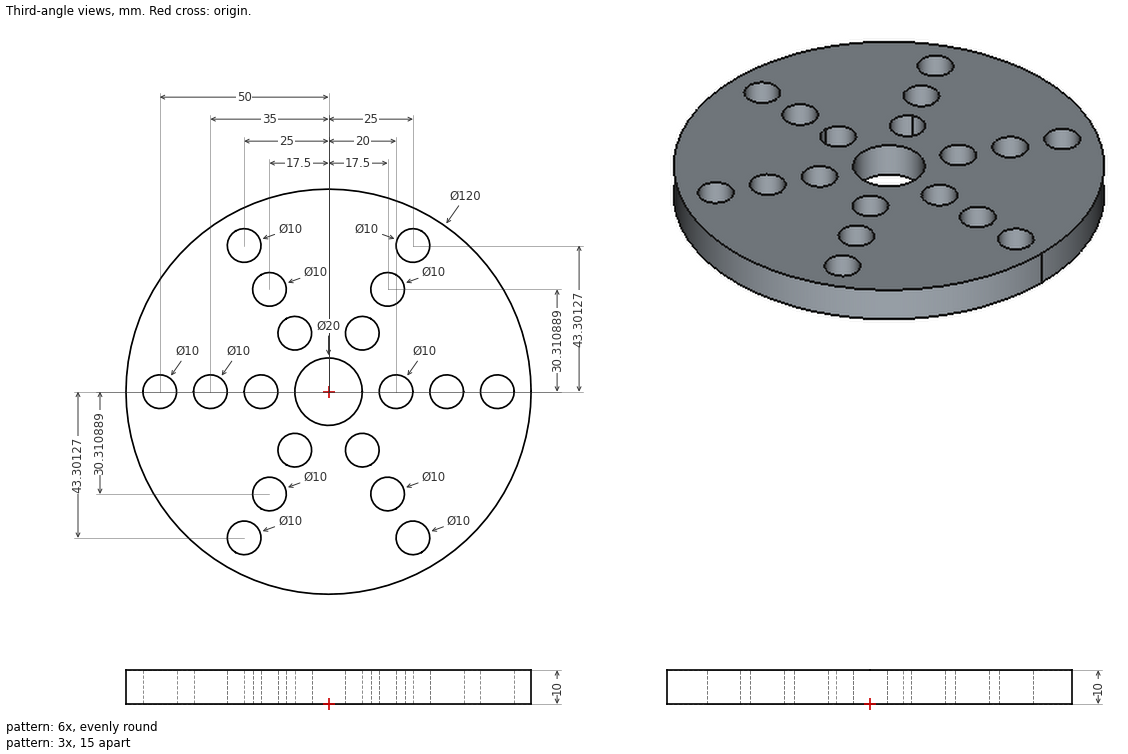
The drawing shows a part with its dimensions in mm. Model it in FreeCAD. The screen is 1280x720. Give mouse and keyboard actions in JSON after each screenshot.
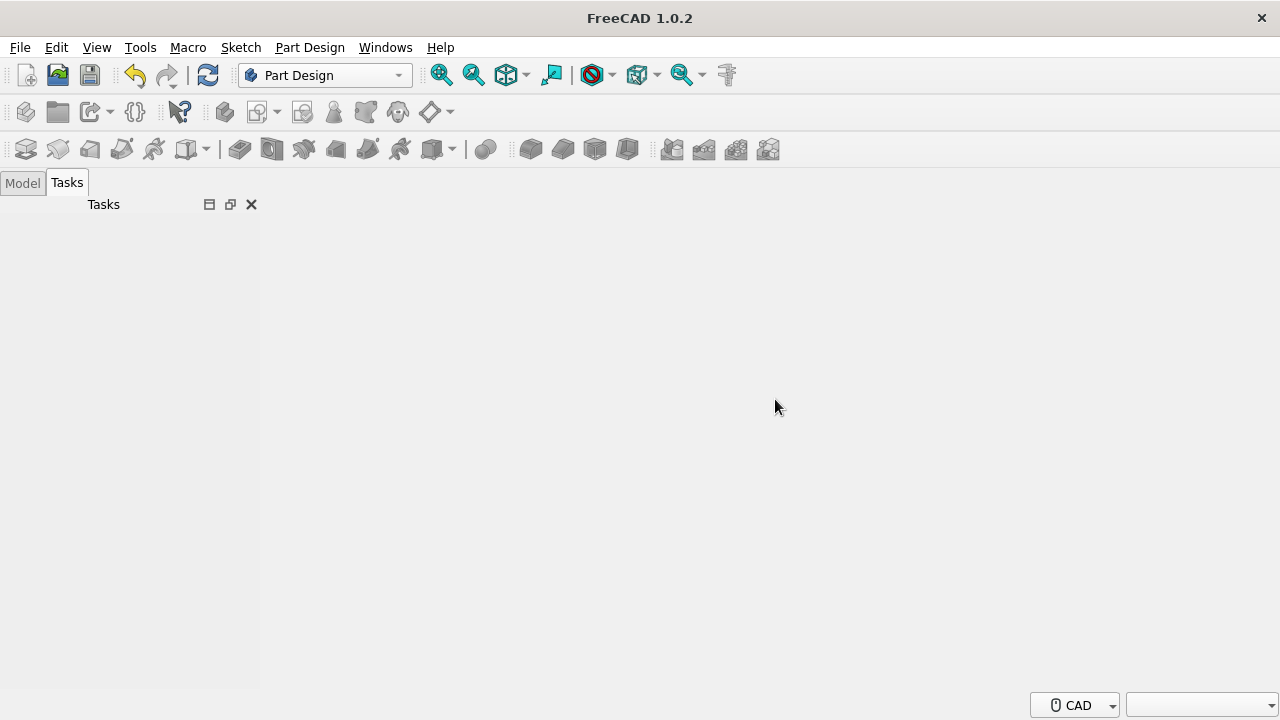
{"action": "key", "text": "ctrl+n"}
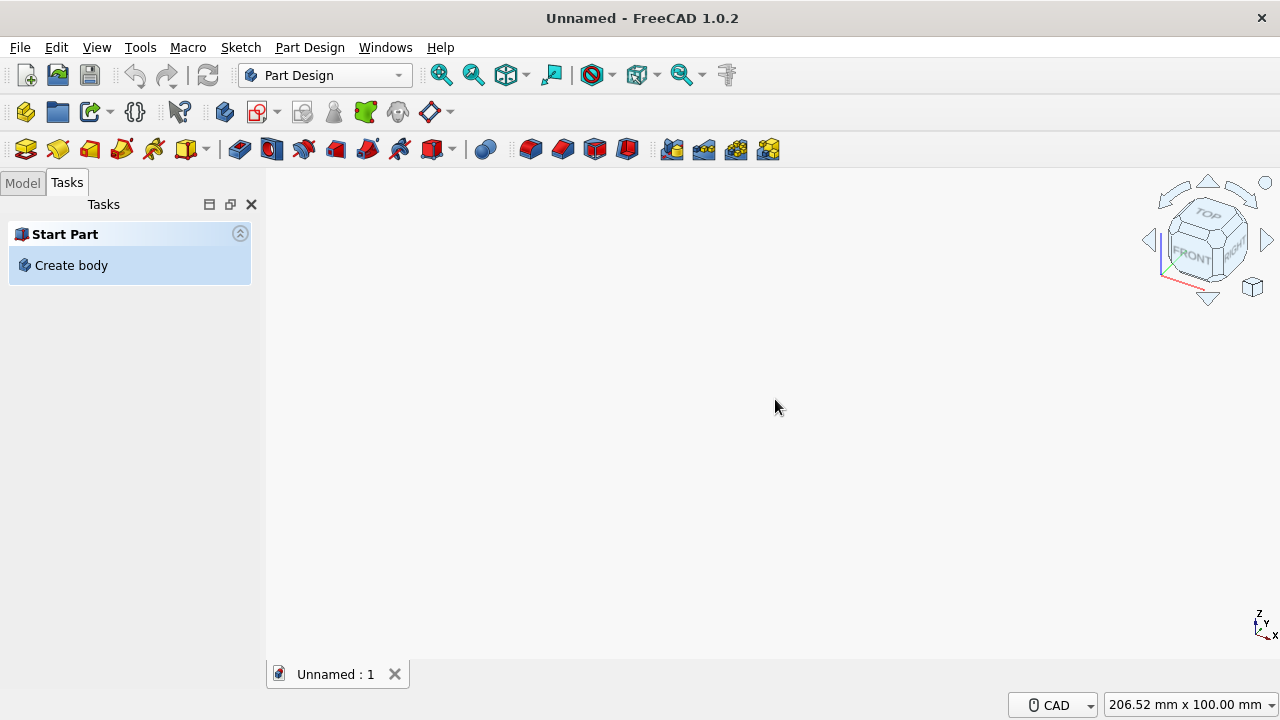
{"action": "left_click", "coordinate": [258, 112]}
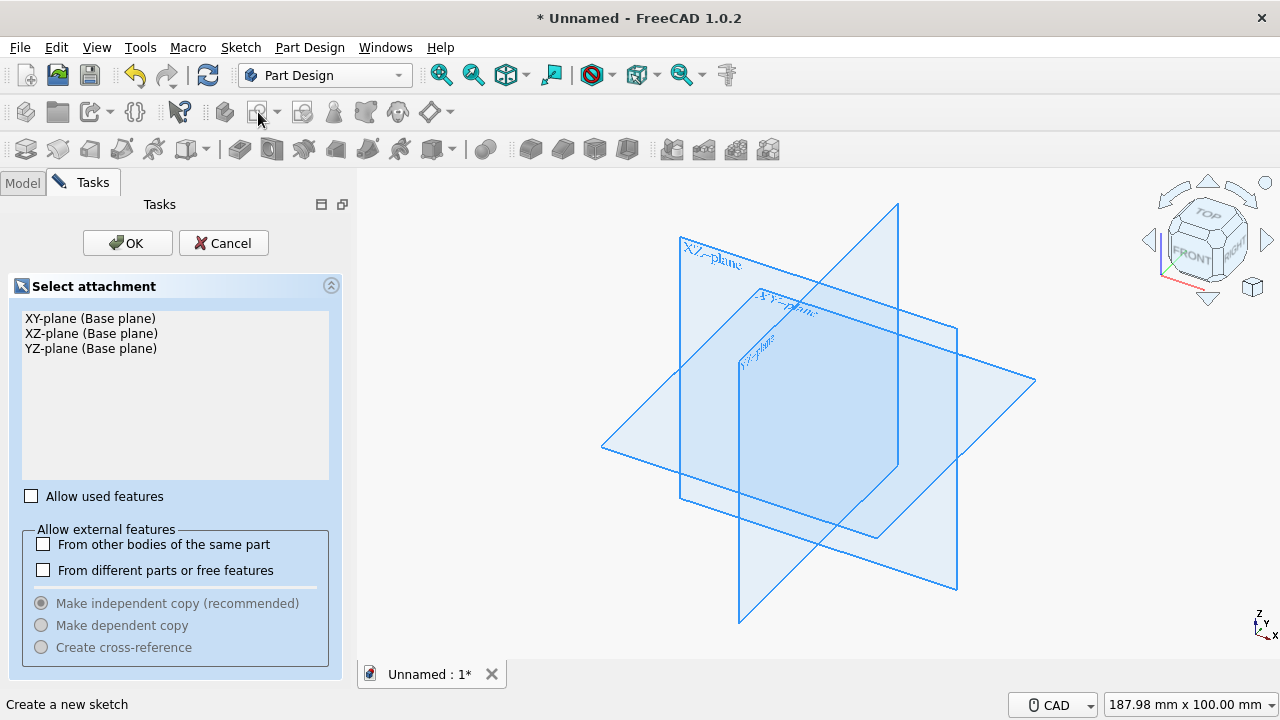
{"action": "left_click", "coordinate": [82, 318]}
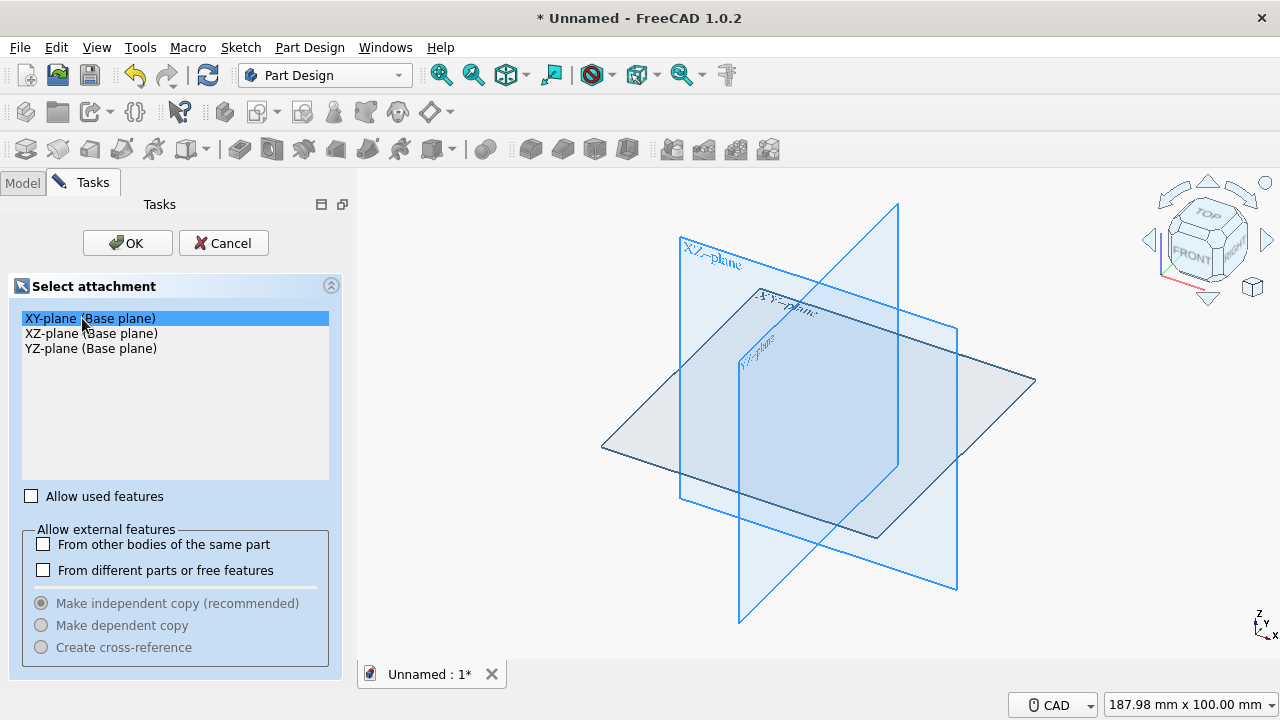
{"action": "left_click", "coordinate": [128, 243]}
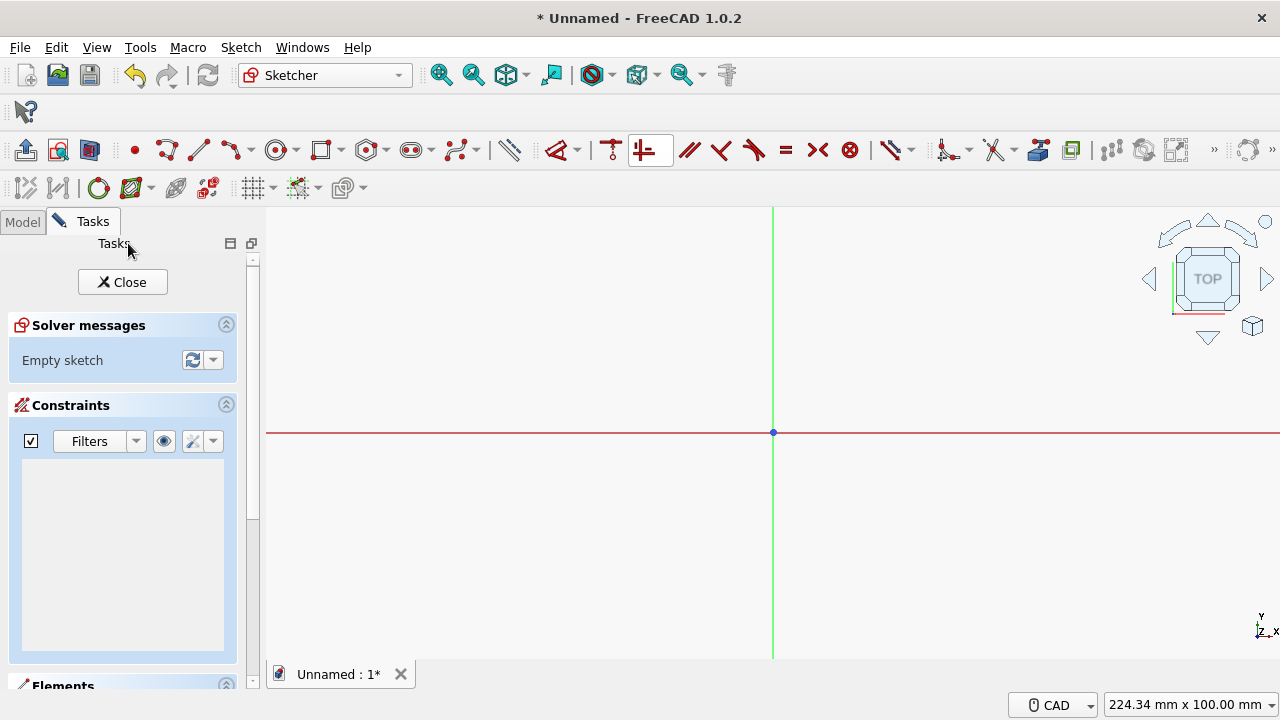
{"action": "scroll", "coordinate": [621, 433], "scroll_direction": "down", "scroll_amount": 3}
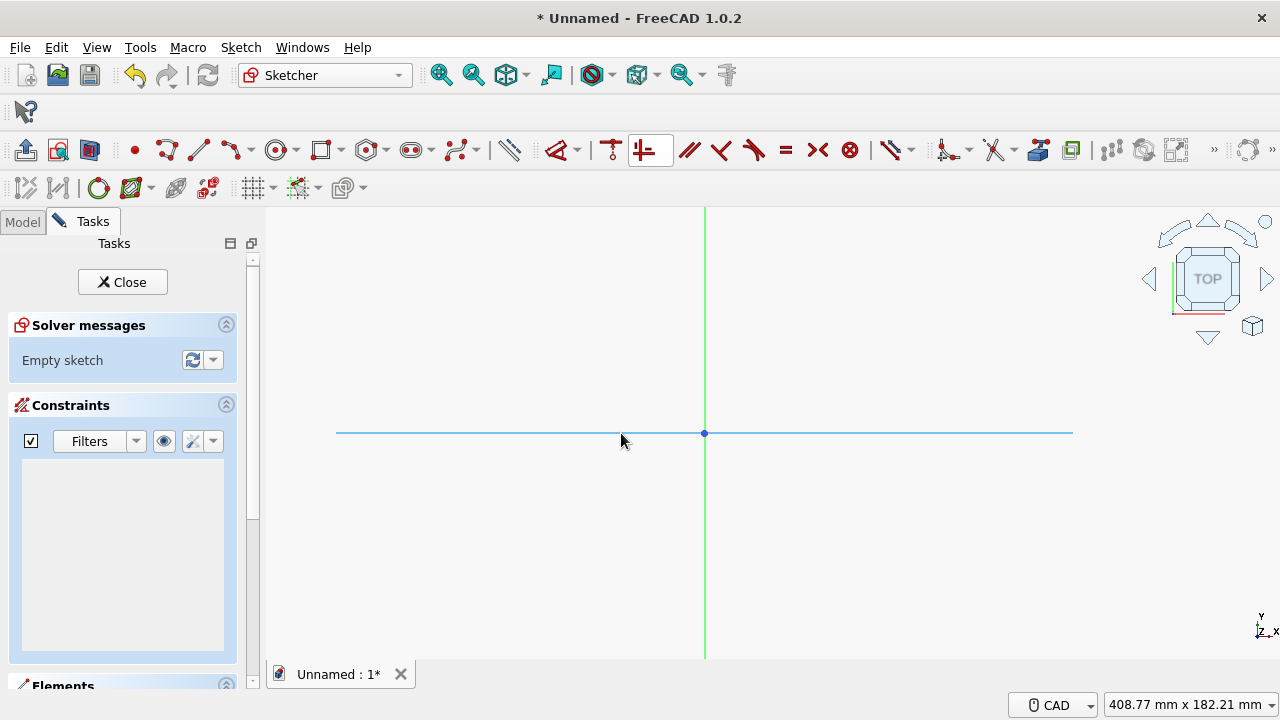
{"action": "left_click", "coordinate": [276, 150]}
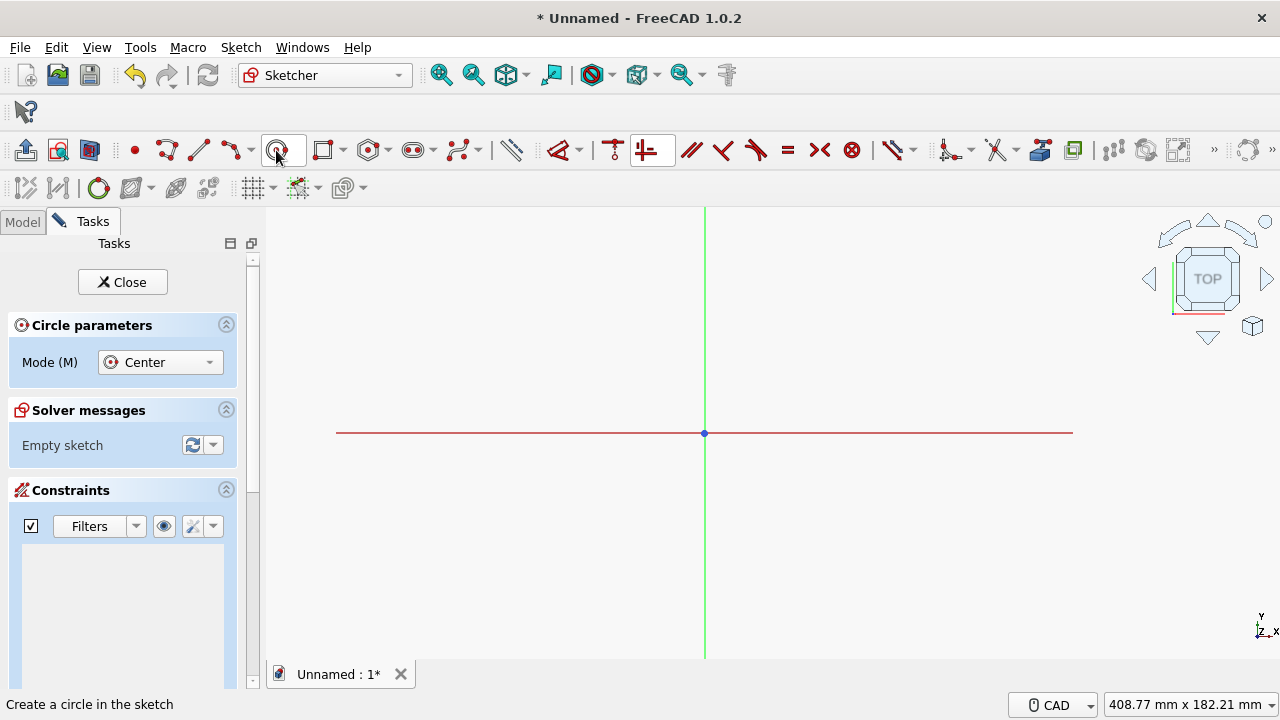
{"action": "left_click", "coordinate": [705, 433]}
{"action": "left_click", "coordinate": [810, 328]}
{"action": "key", "text": "Escape"}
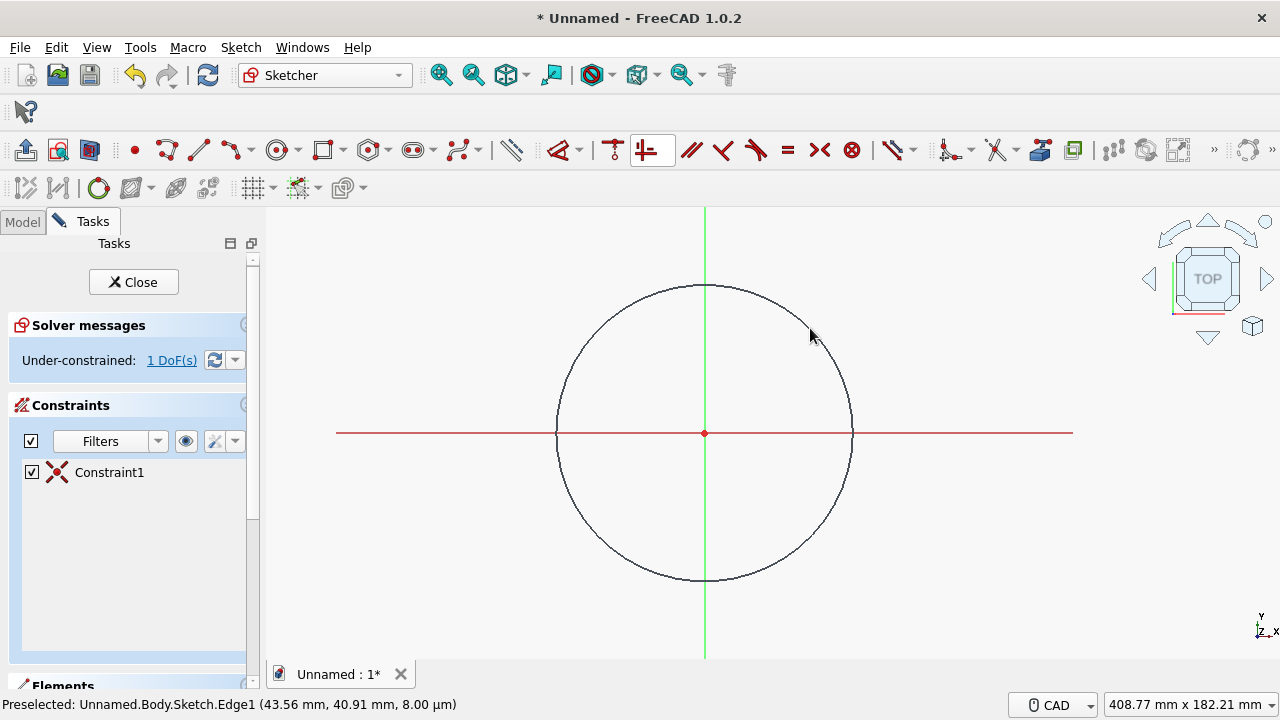
{"action": "key", "text": "d"}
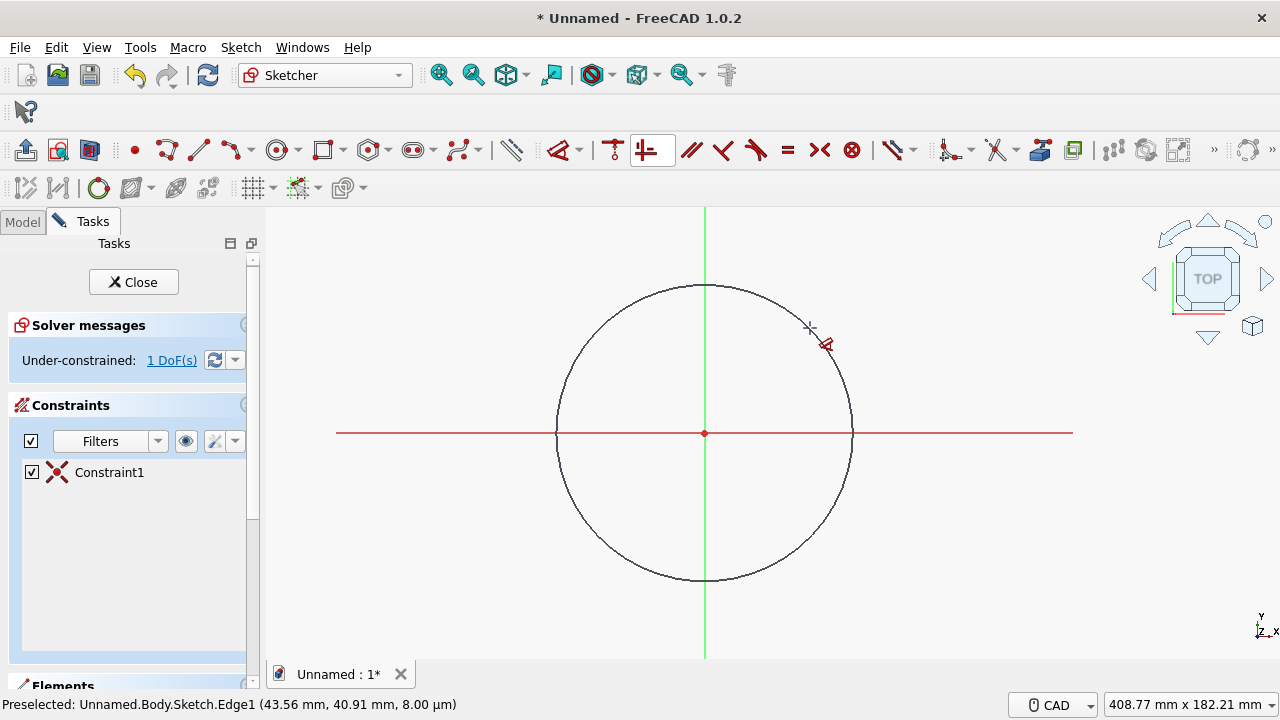
{"action": "left_click", "coordinate": [809, 328]}
{"action": "left_click", "coordinate": [832, 305]}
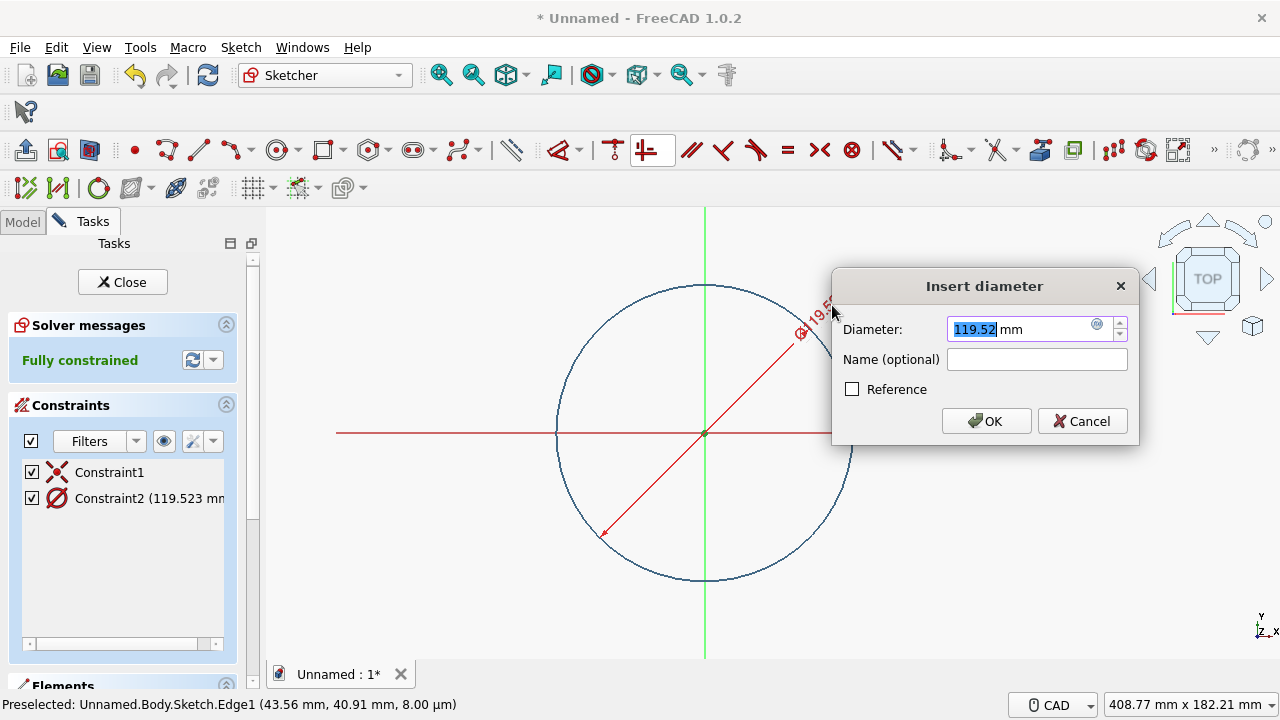
{"action": "type", "text": "120"}
{"action": "key", "text": "Return"}
{"action": "key", "text": "Escape"}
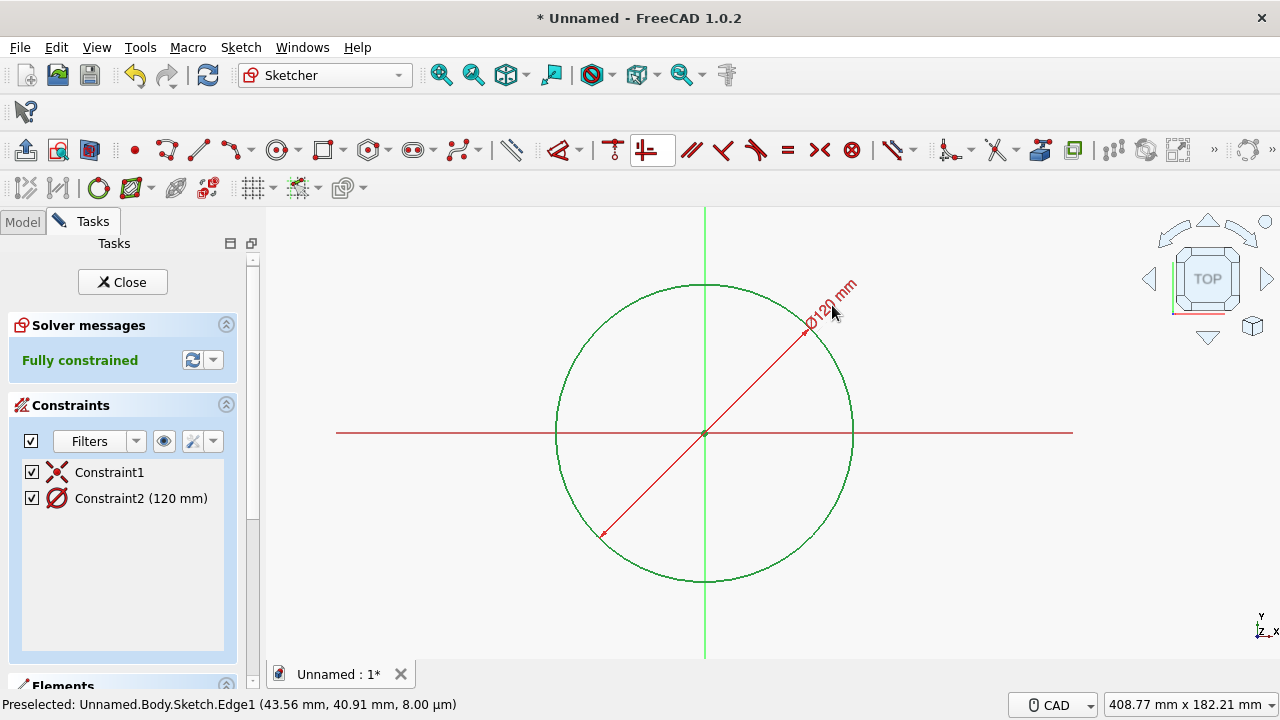
{"action": "left_click", "coordinate": [123, 282]}